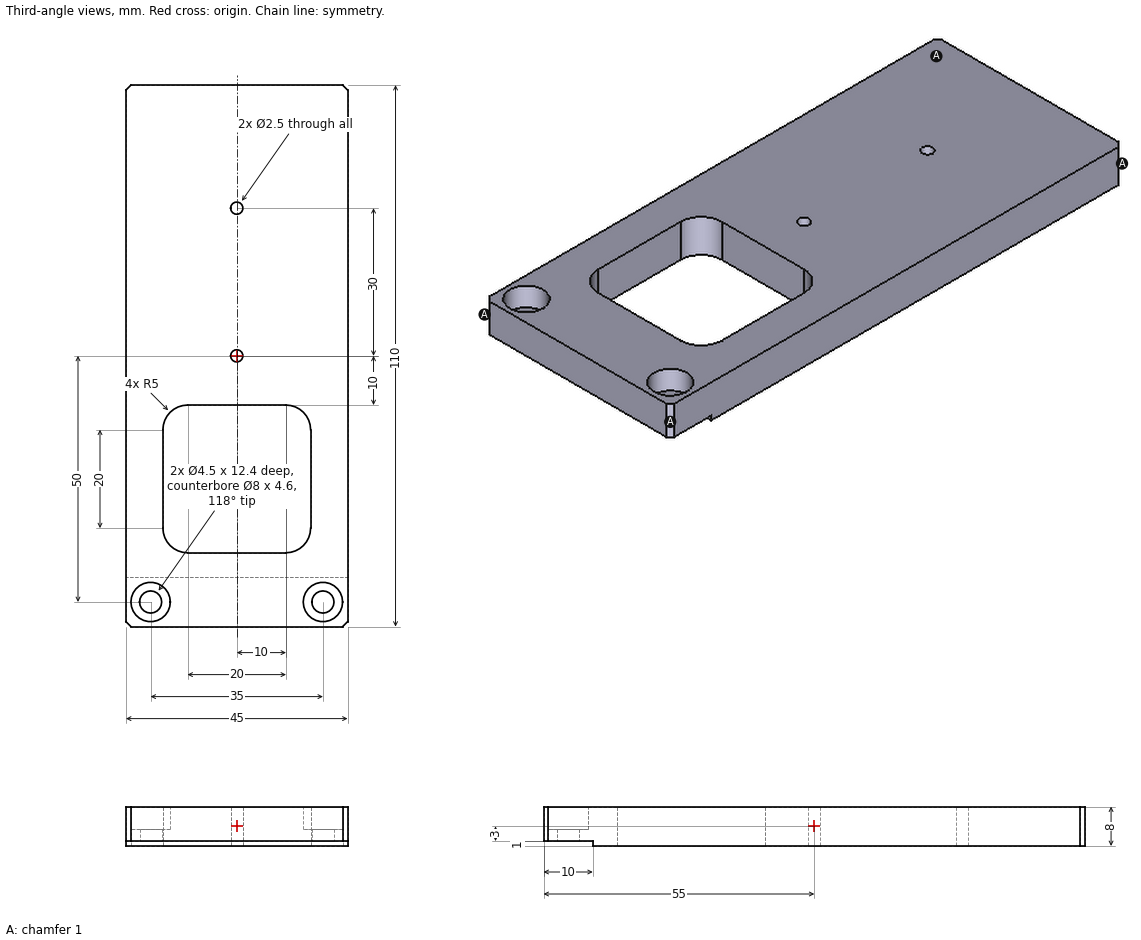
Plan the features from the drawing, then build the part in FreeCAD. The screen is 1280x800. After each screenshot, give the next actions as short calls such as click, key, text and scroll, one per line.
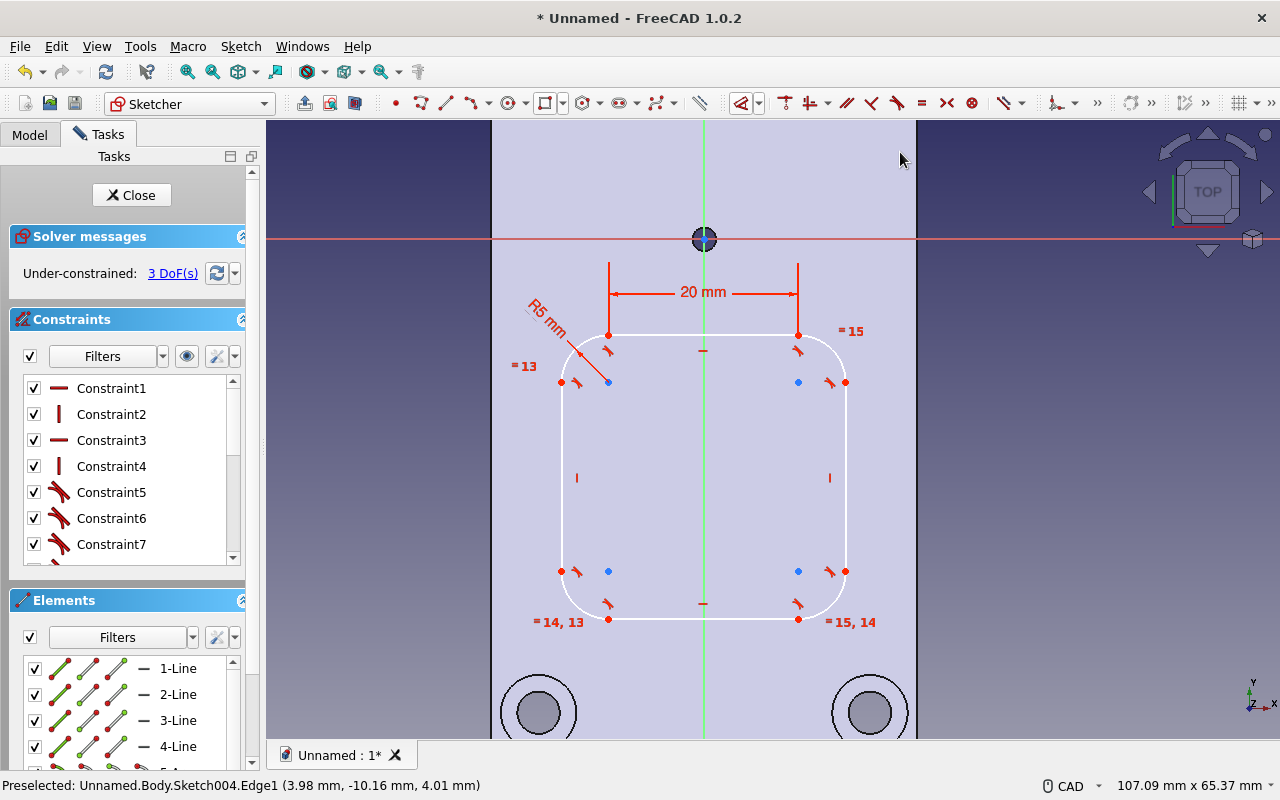
click(562, 439)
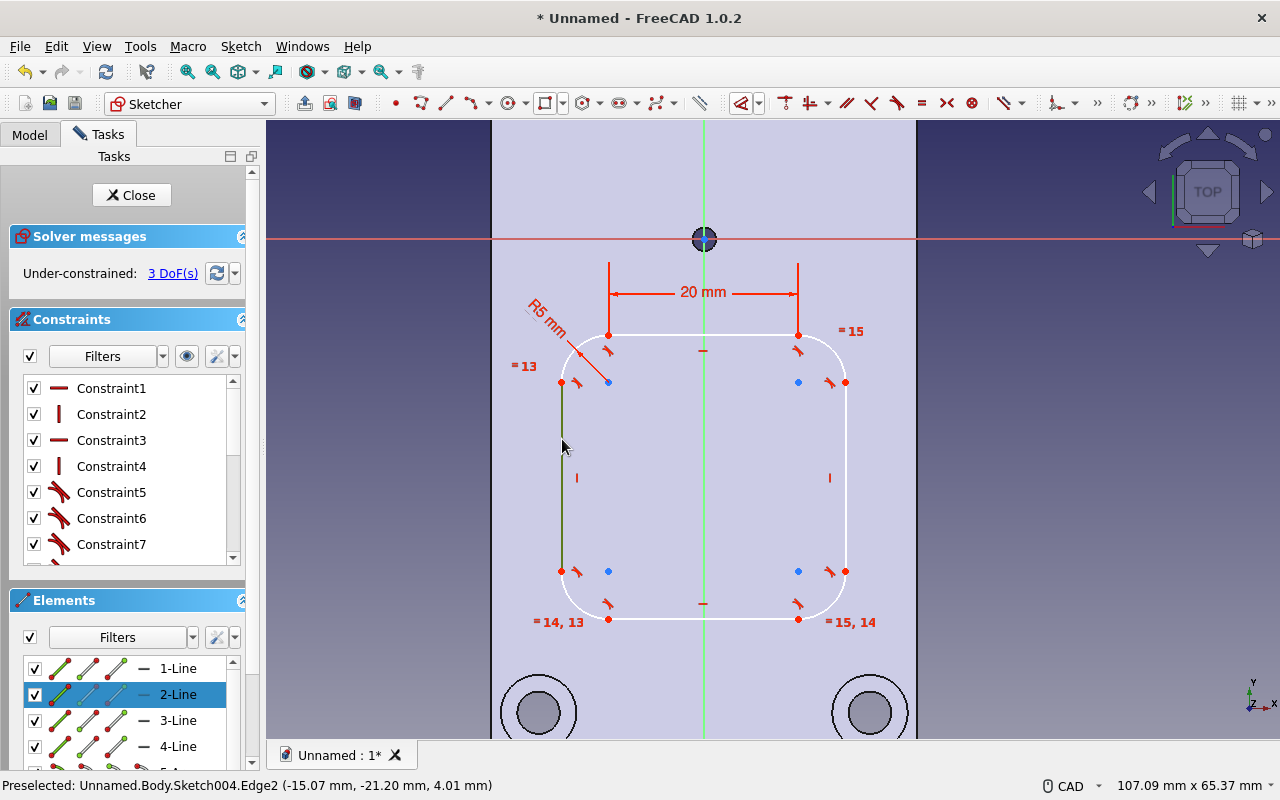
click(758, 104)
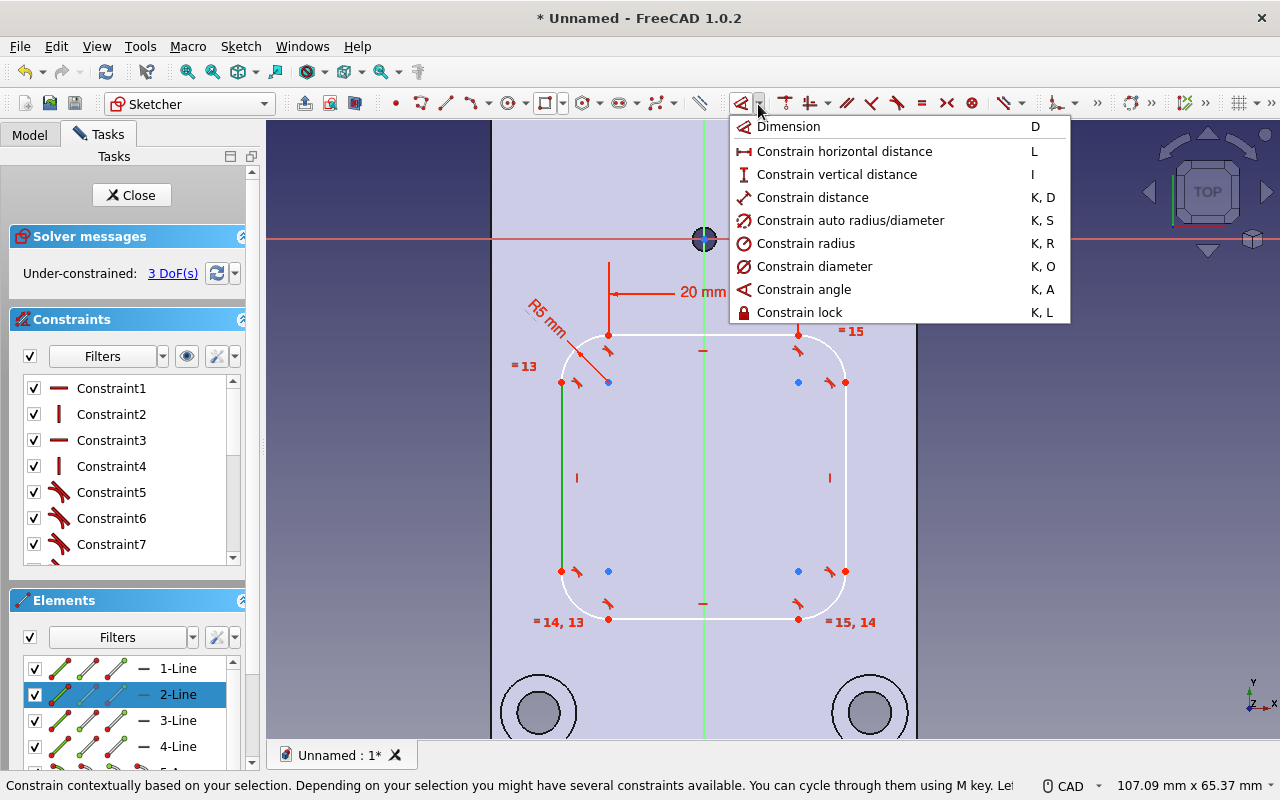
click(900, 174)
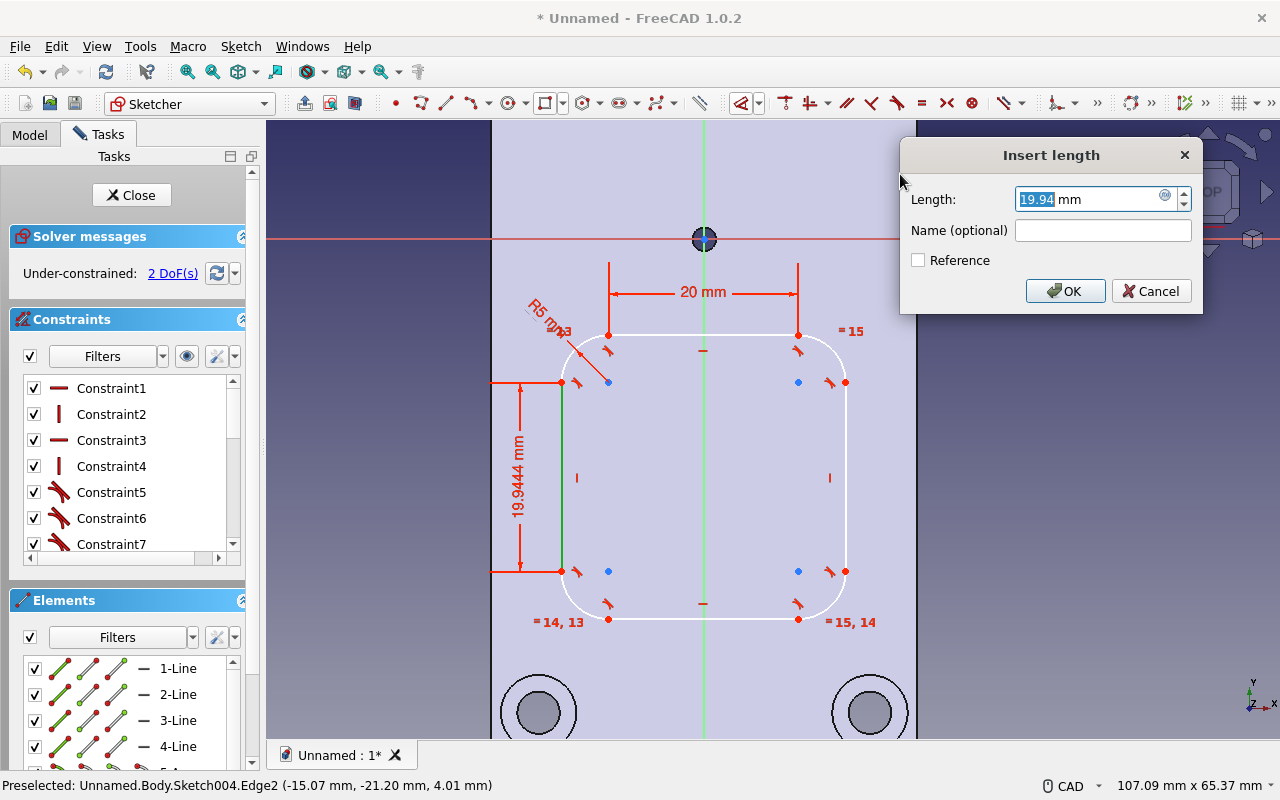
text(20)
key(Return)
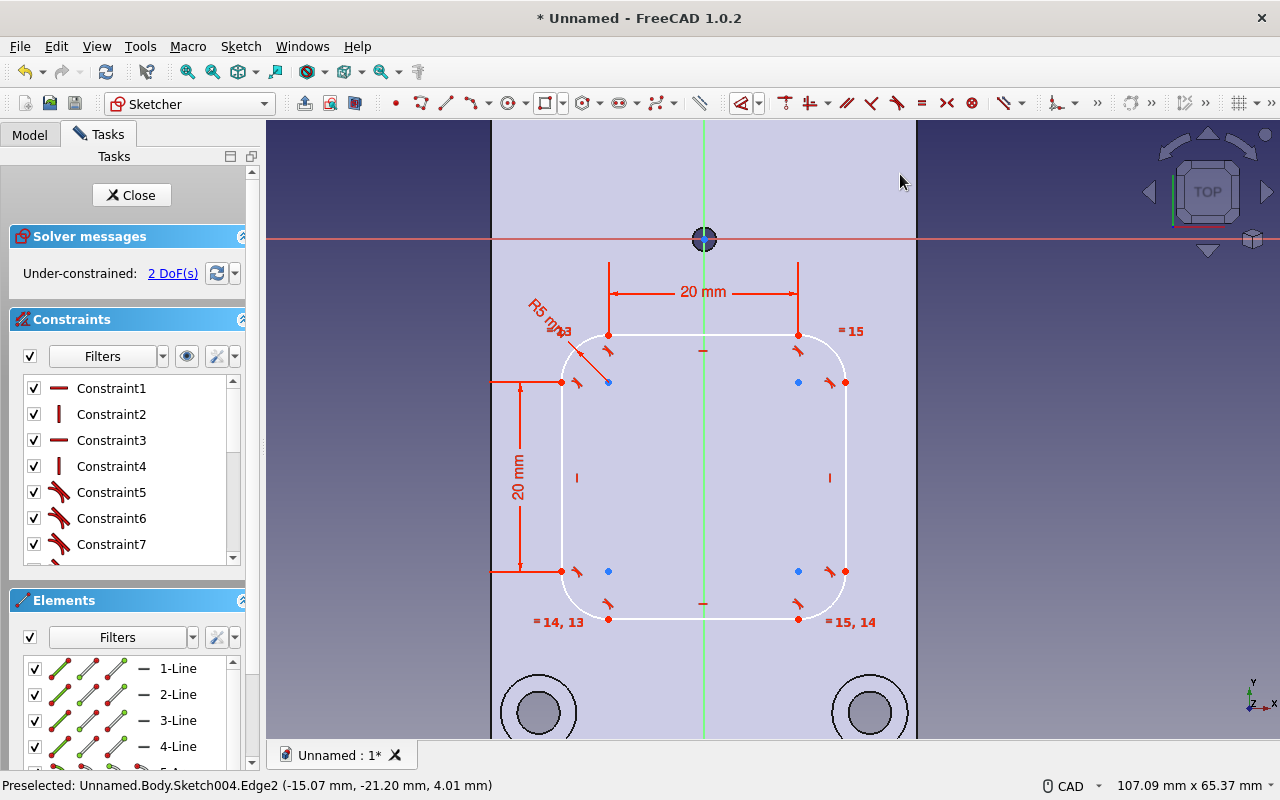
click(798, 335)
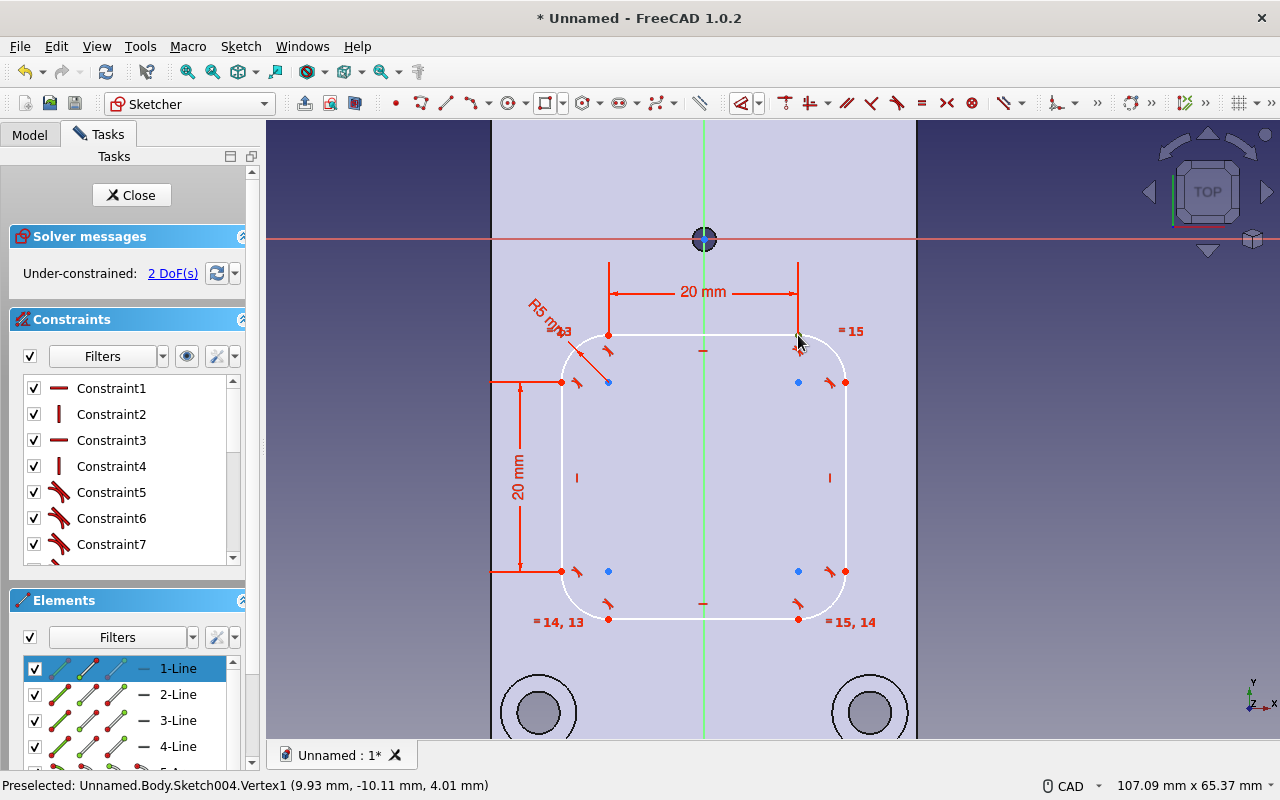
click(758, 104)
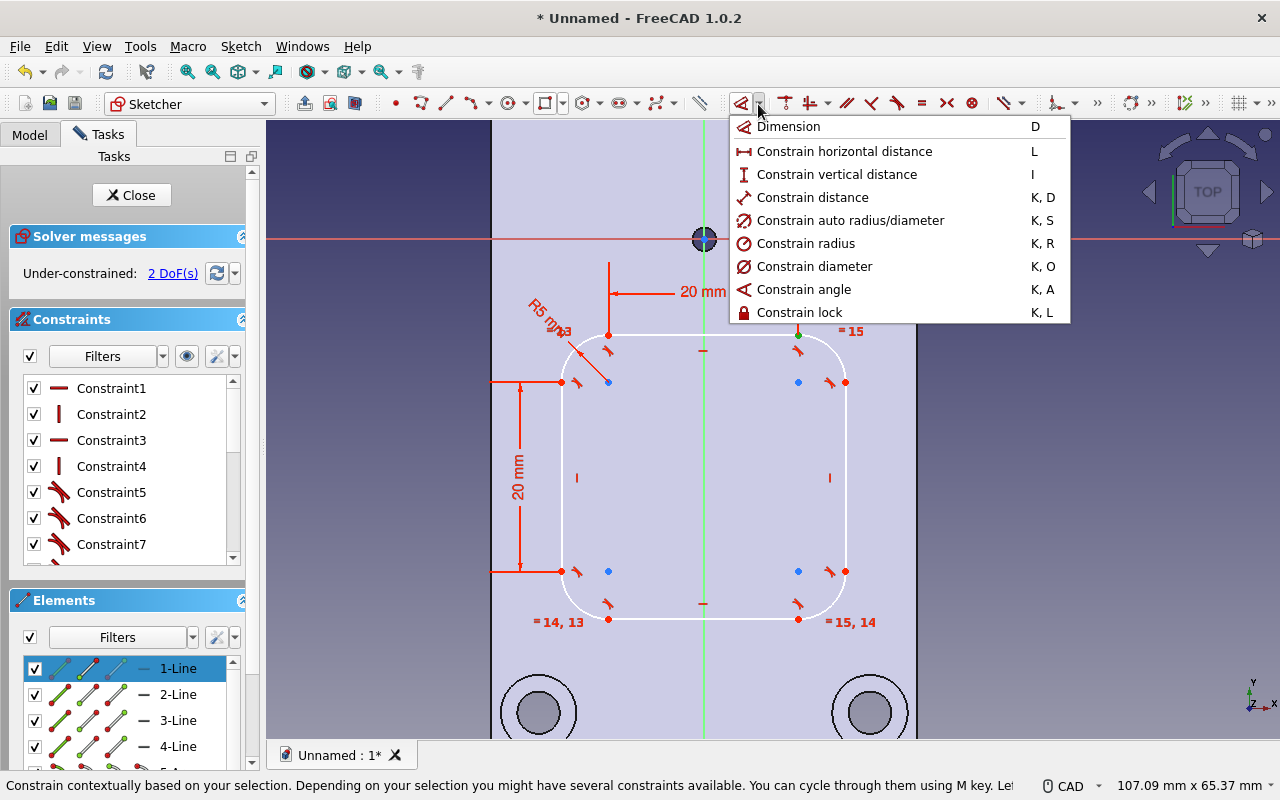
click(900, 152)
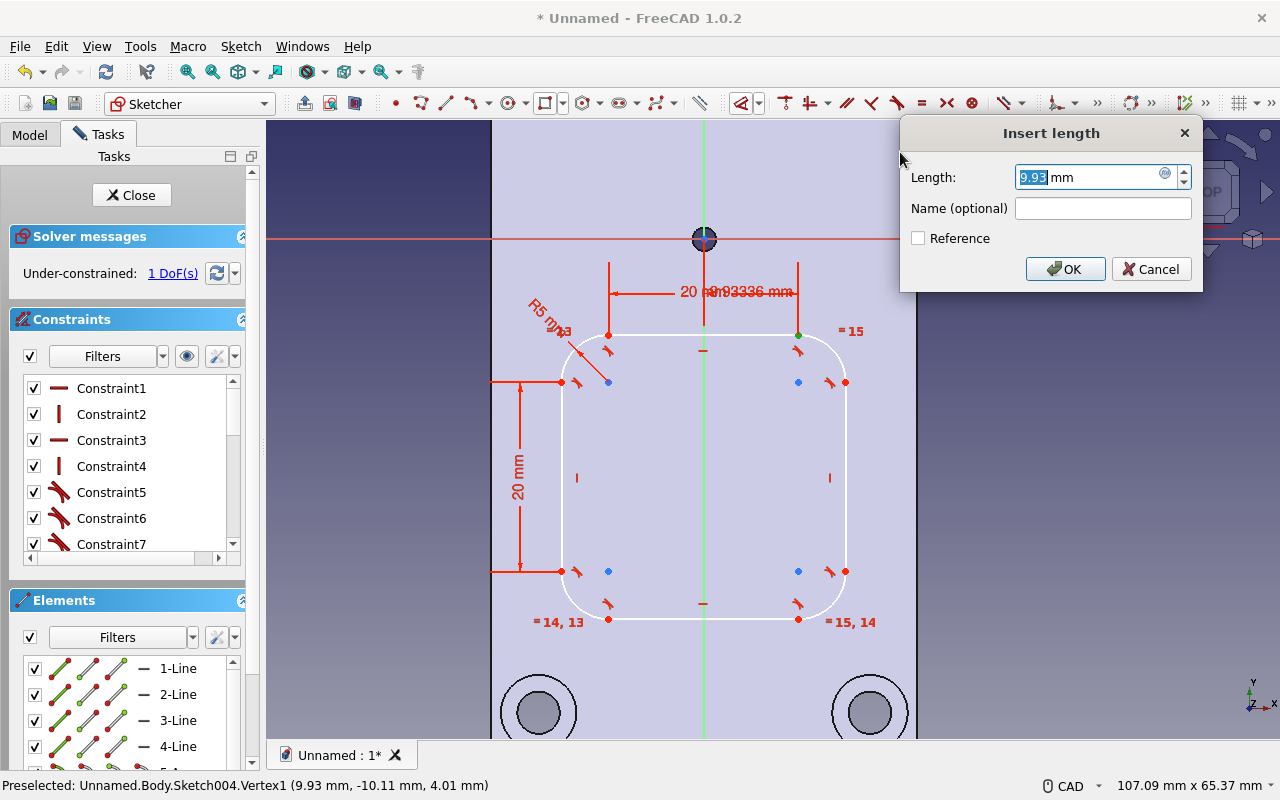
text(10)
key(Return)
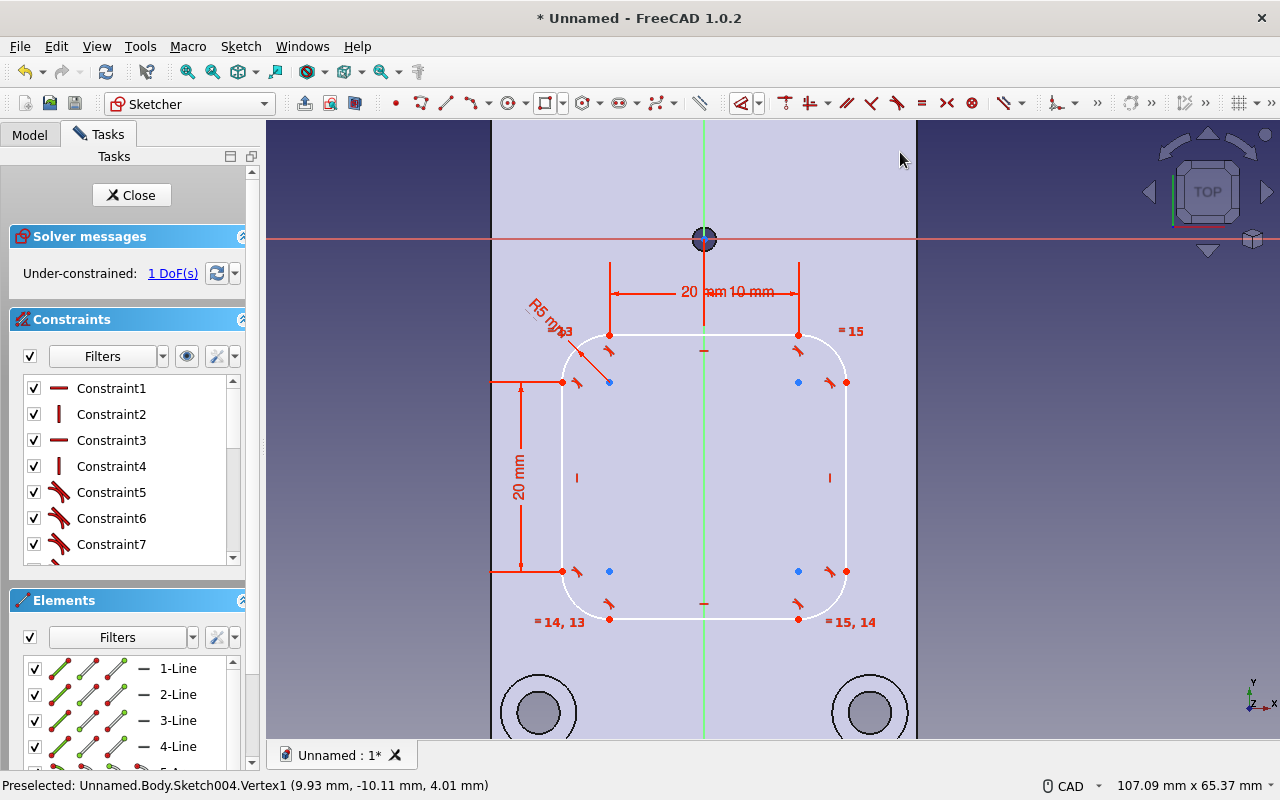
click(799, 335)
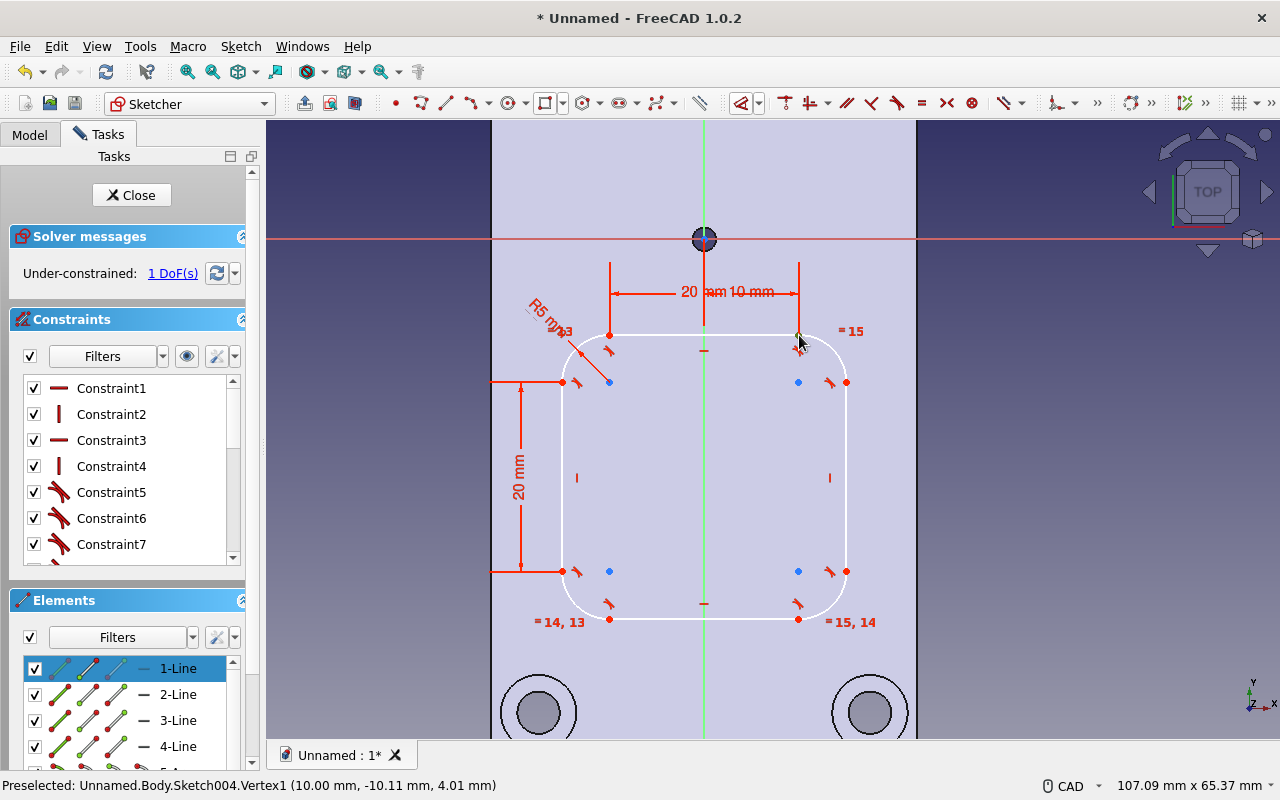
click(758, 104)